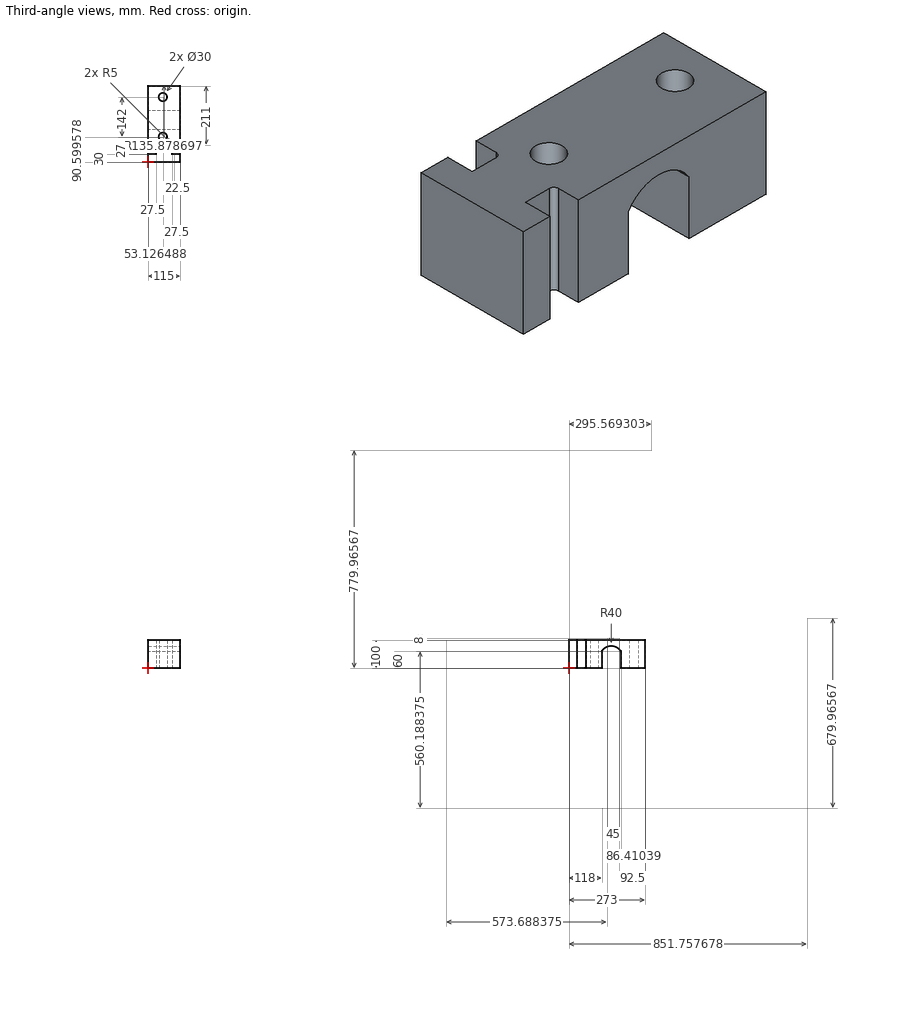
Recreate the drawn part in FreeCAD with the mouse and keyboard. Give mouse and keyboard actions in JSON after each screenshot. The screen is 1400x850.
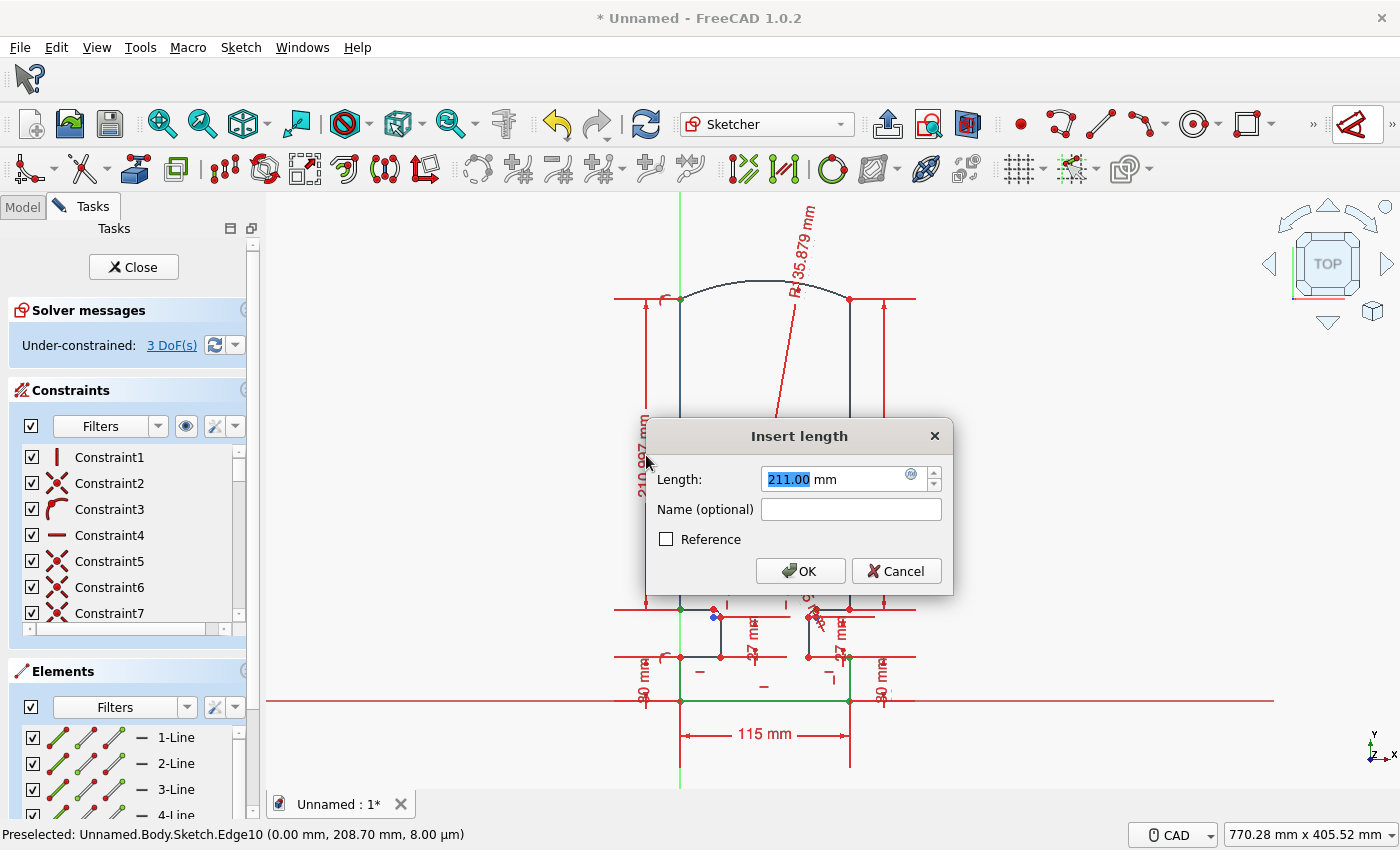
{"action": "type", "text": "211"}
{"action": "key", "text": "Return"}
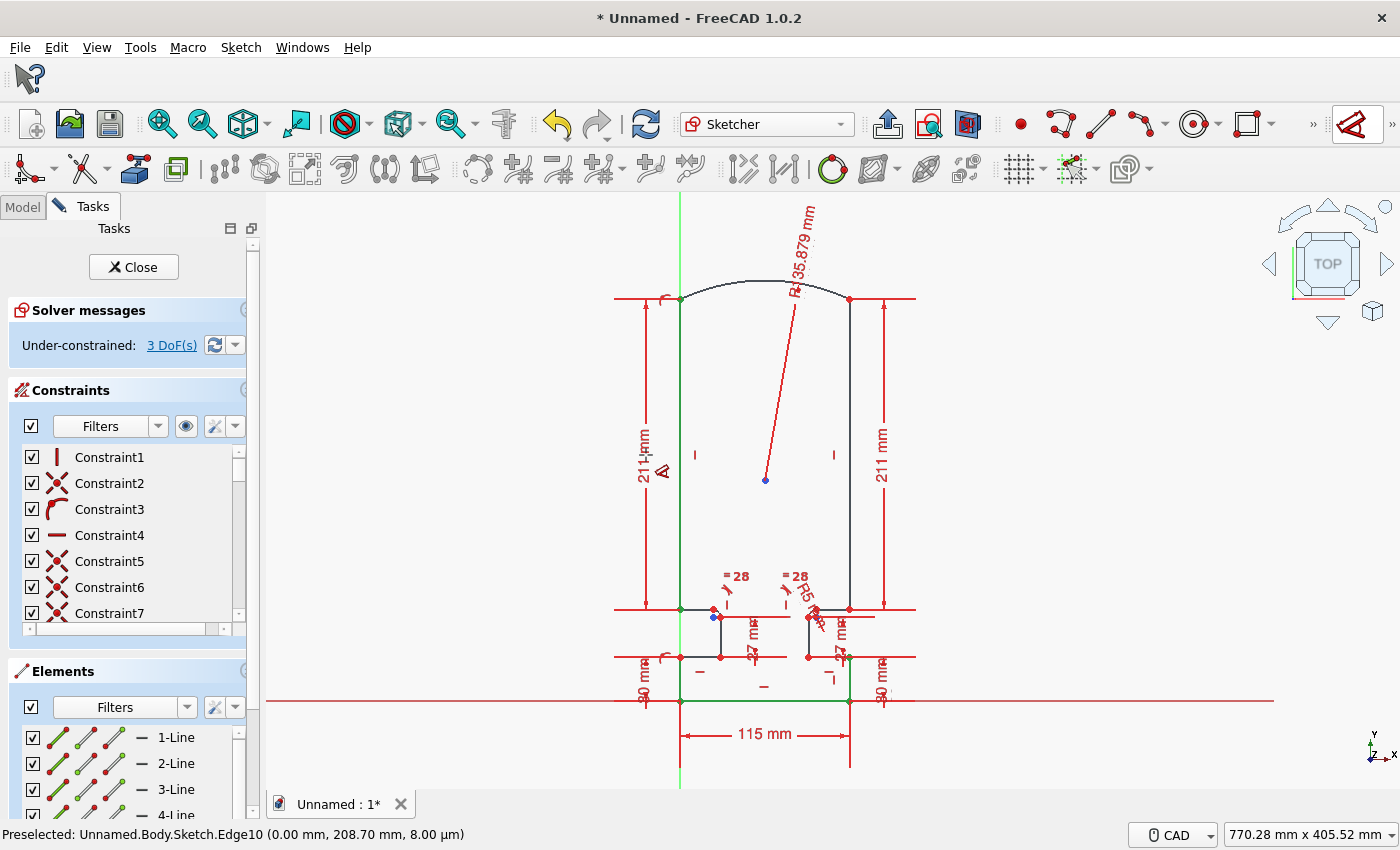
{"action": "left_click", "coordinate": [709, 657]}
{"action": "left_click", "coordinate": [701, 715]}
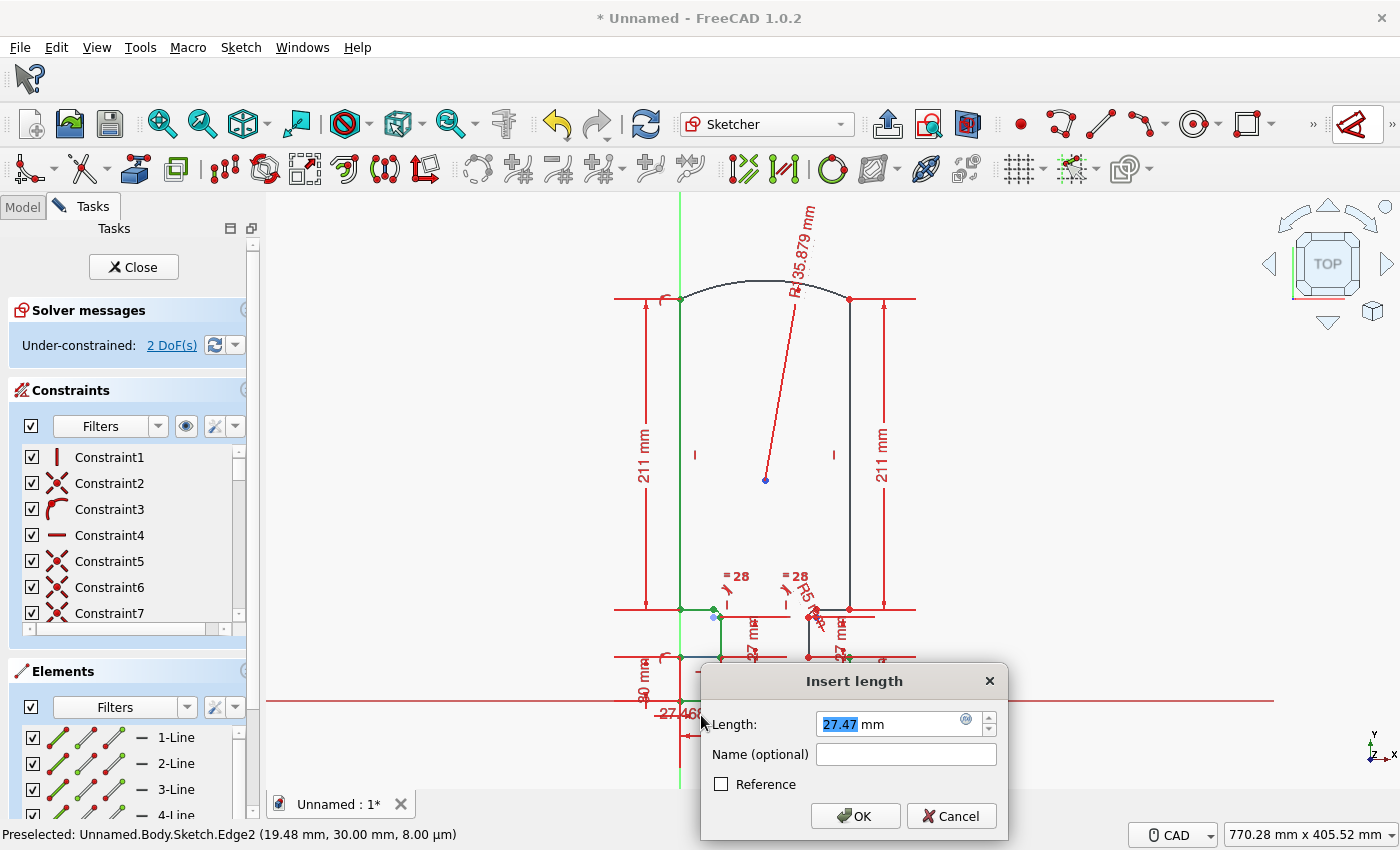
{"action": "type", "text": "27.5"}
{"action": "key", "text": "Return"}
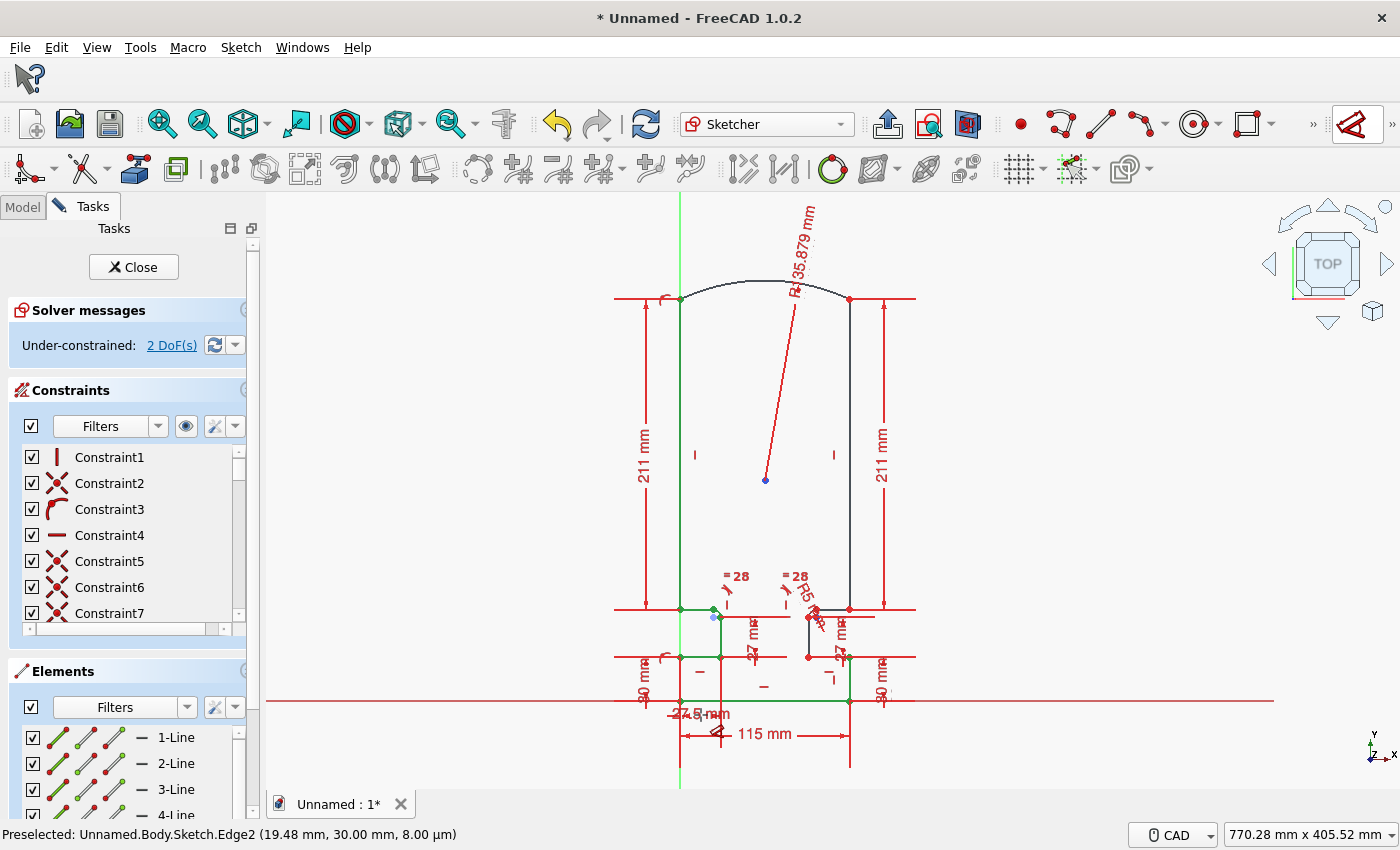
{"action": "left_click", "coordinate": [837, 657]}
{"action": "left_click", "coordinate": [829, 715]}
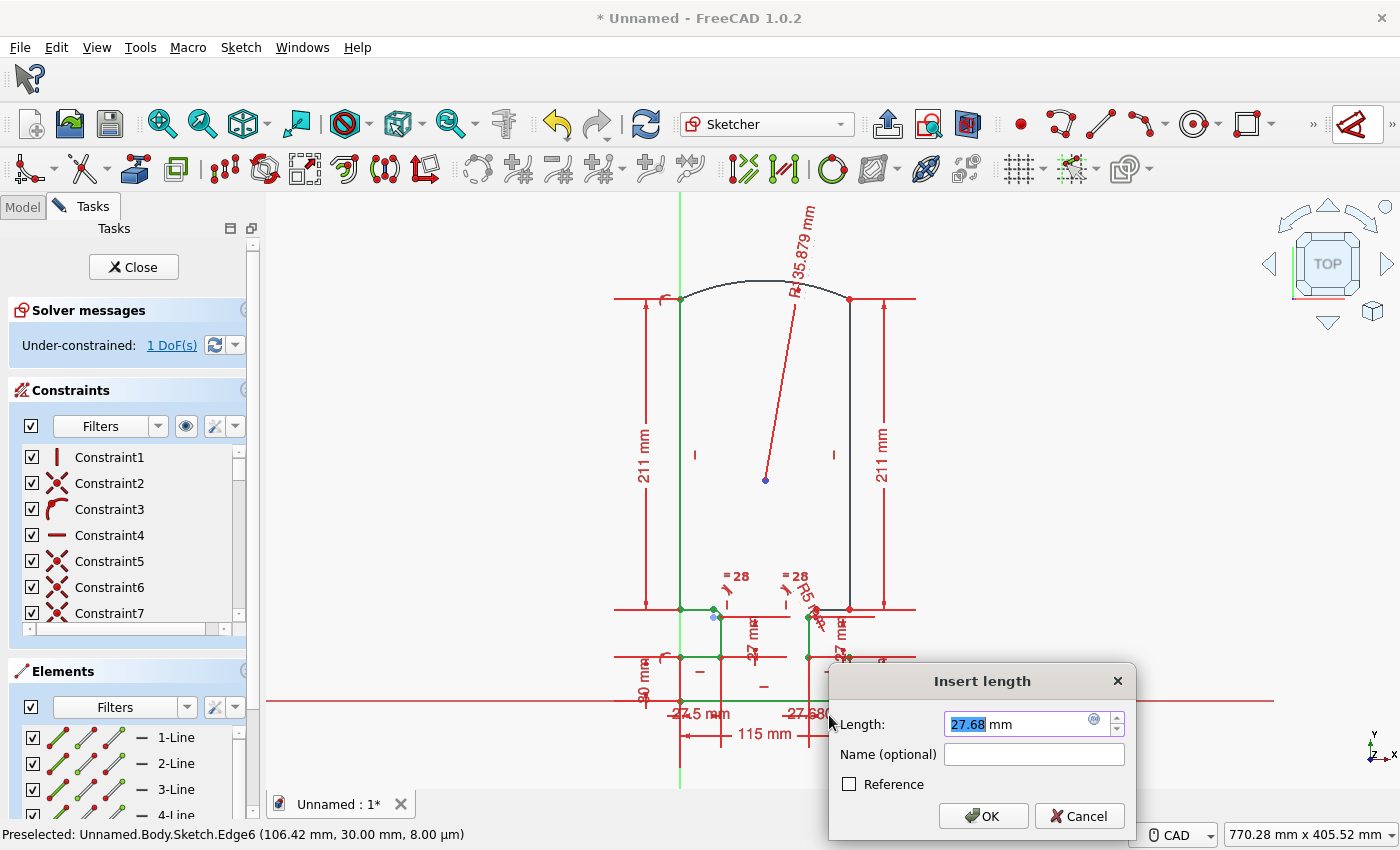
{"action": "type", "text": "27.5"}
{"action": "key", "text": "Return"}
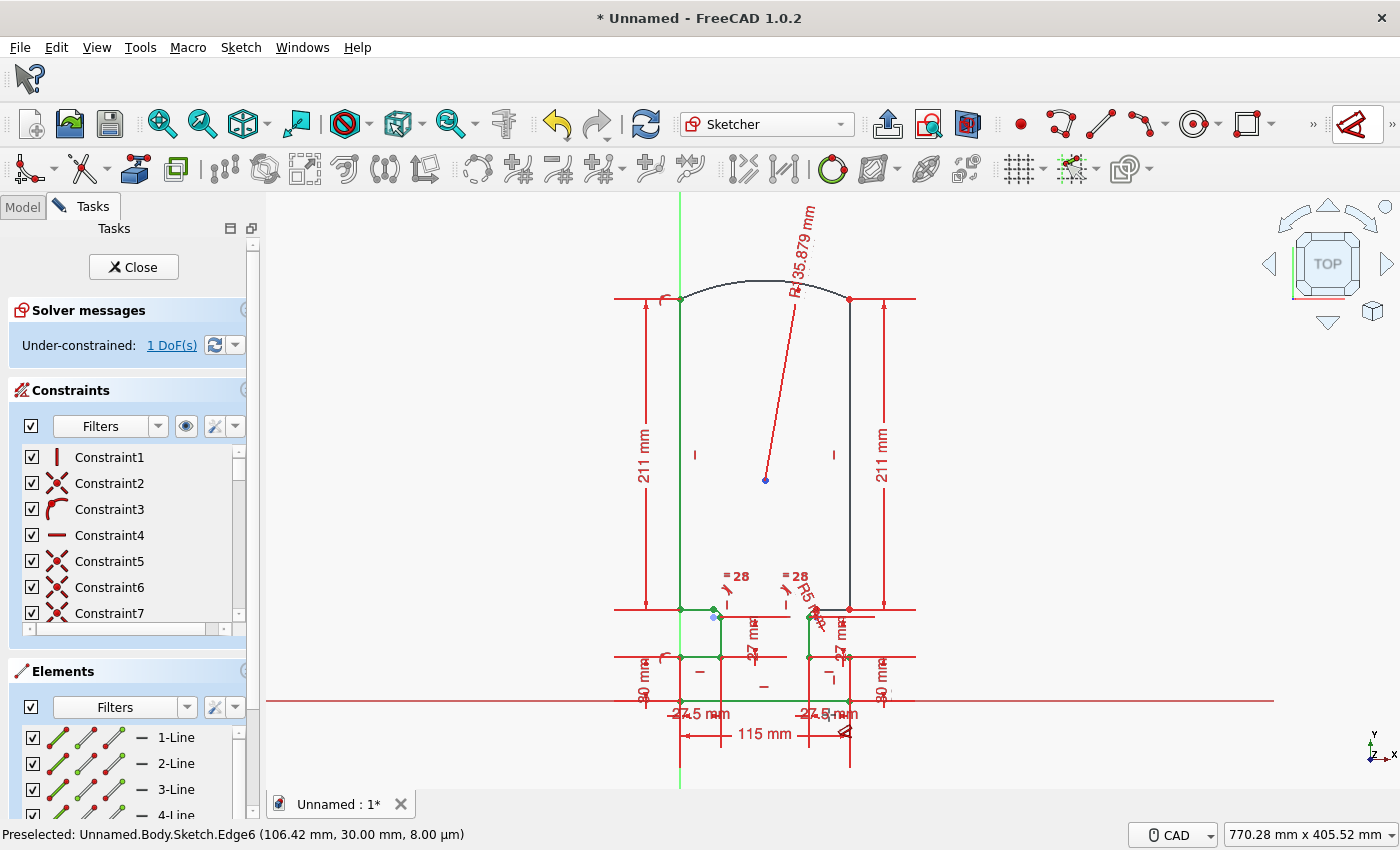
{"action": "scroll", "coordinate": [826, 610], "scroll_direction": "up", "scroll_amount": 2}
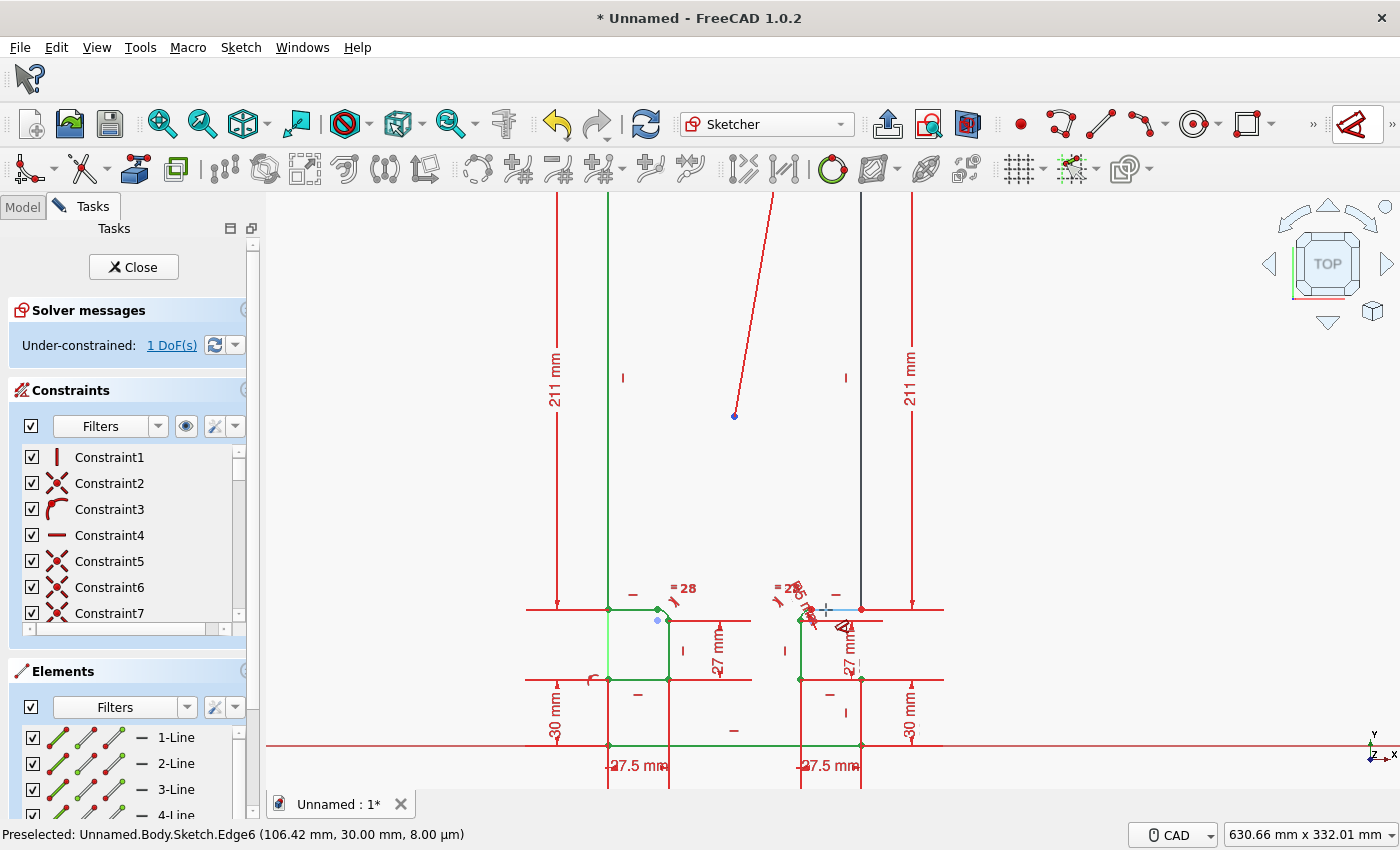
{"action": "left_click", "coordinate": [826, 610]}
{"action": "left_click", "coordinate": [836, 576]}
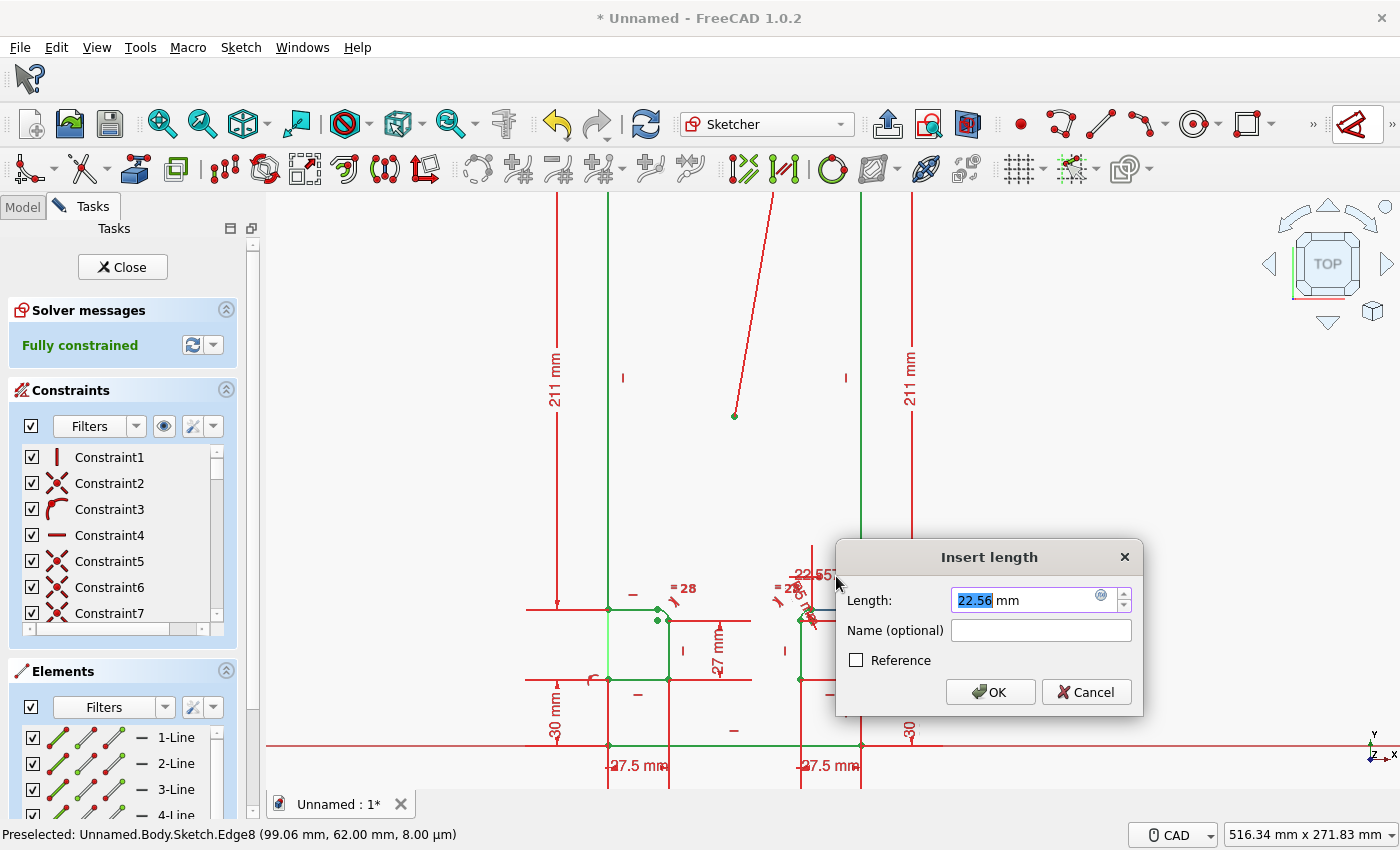
{"action": "type", "text": "22.5"}
{"action": "key", "text": "Return"}
{"action": "key", "text": "Escape"}